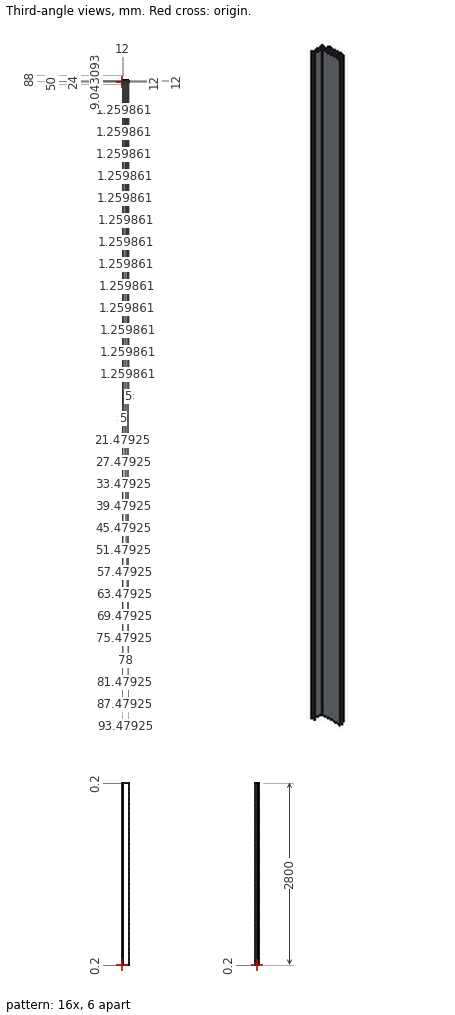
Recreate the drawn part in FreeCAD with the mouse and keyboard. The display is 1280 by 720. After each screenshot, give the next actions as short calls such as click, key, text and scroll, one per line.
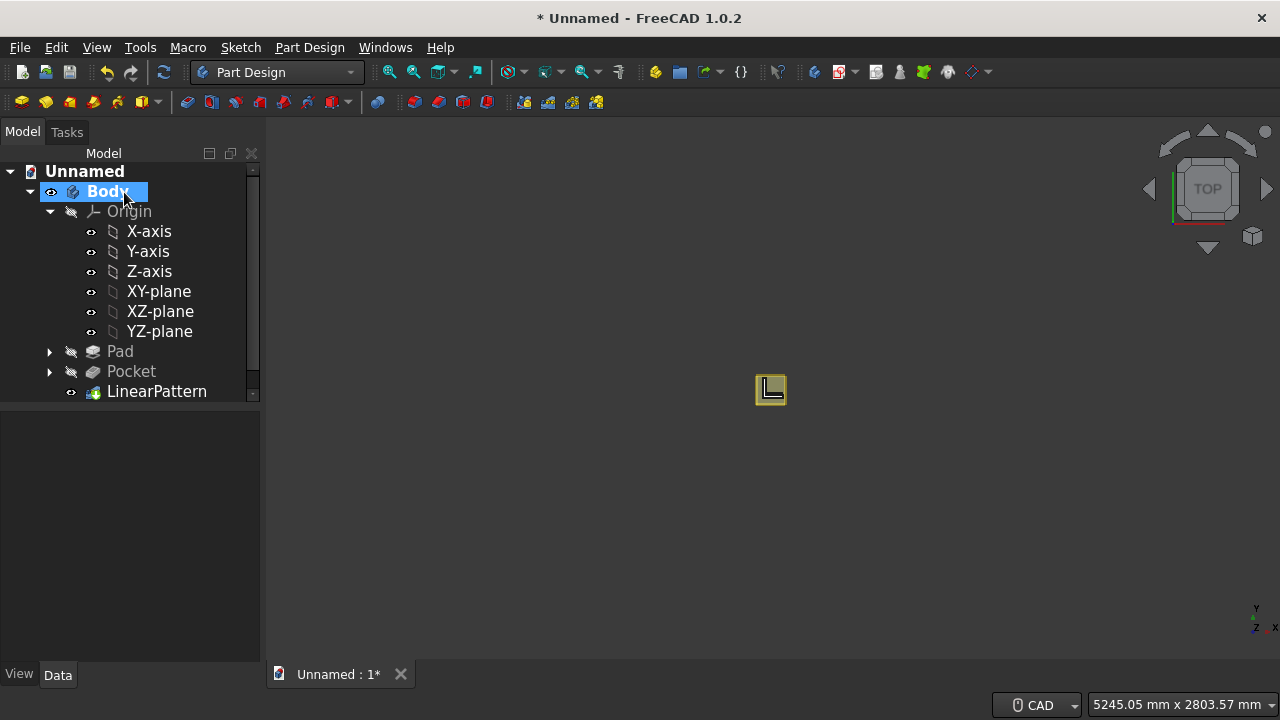
click(116, 372)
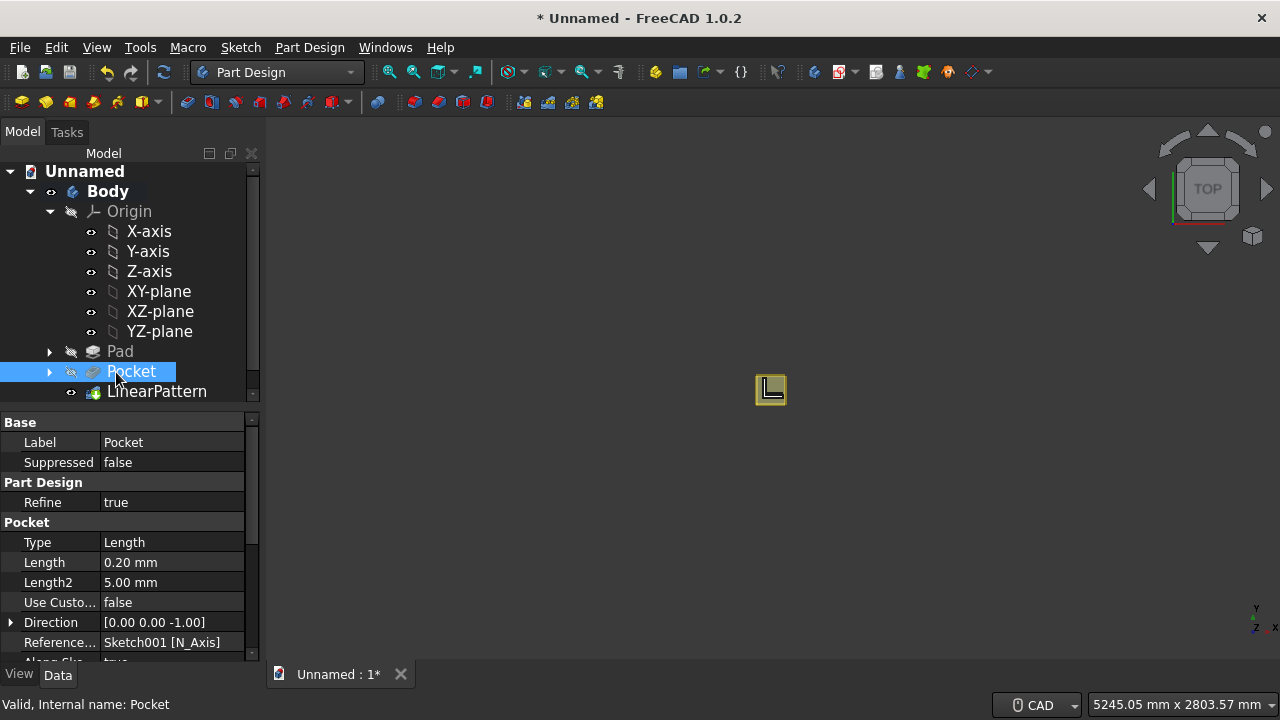
click(524, 102)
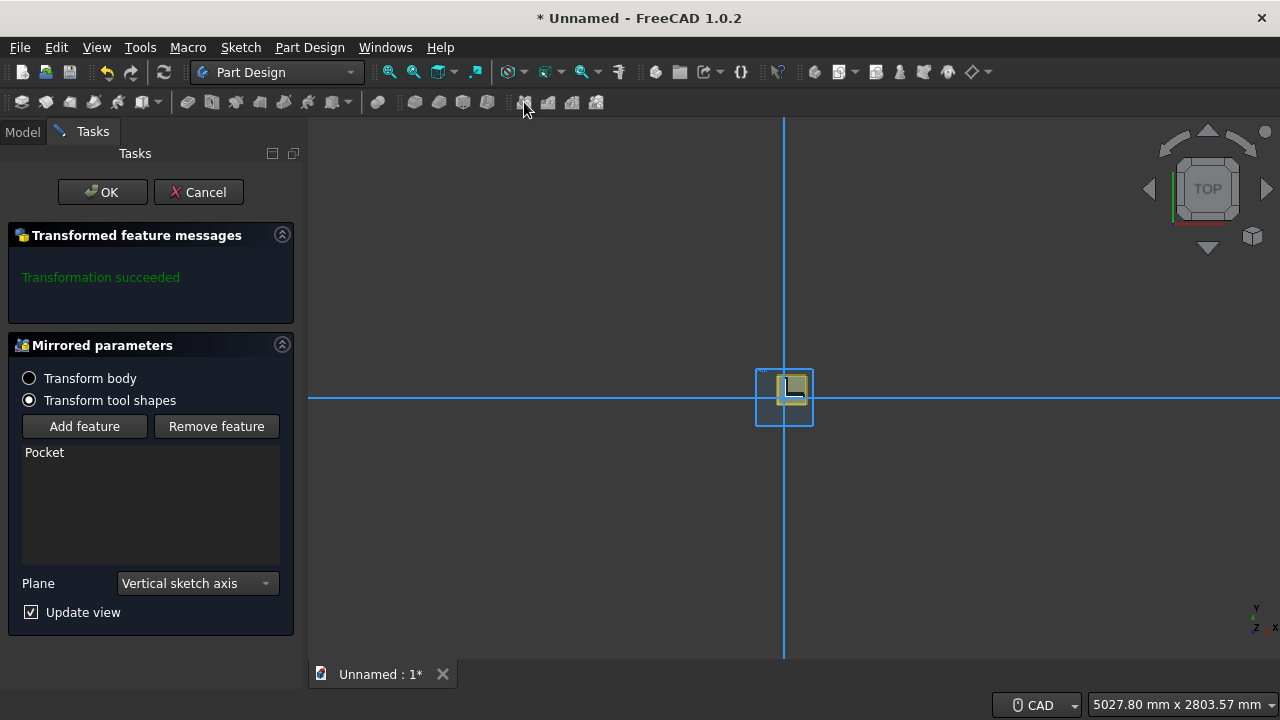
click(198, 584)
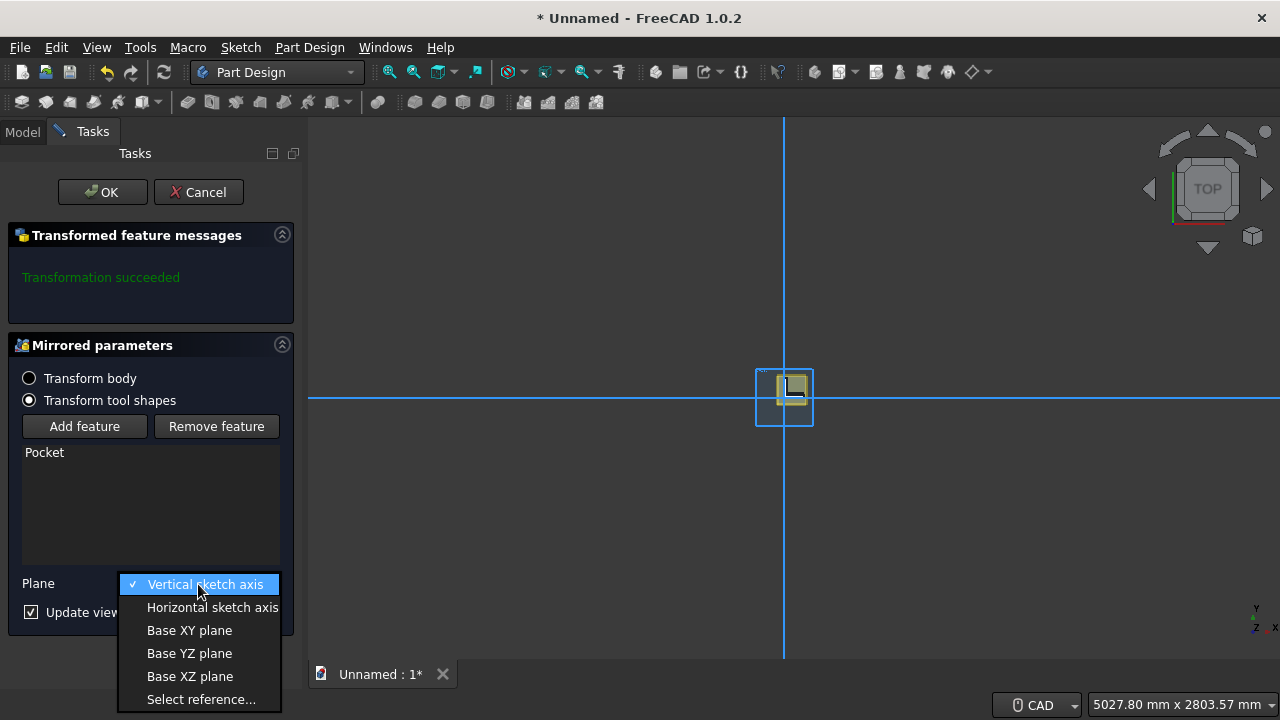
click(198, 700)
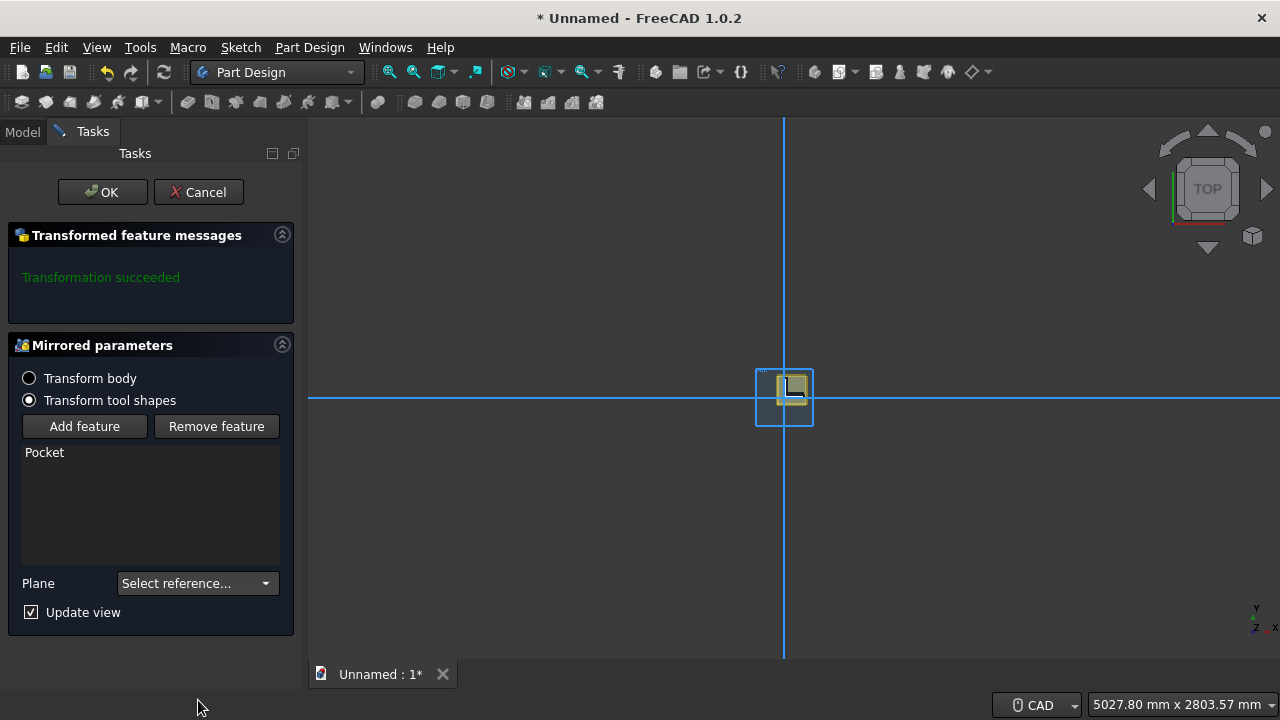
click(23, 131)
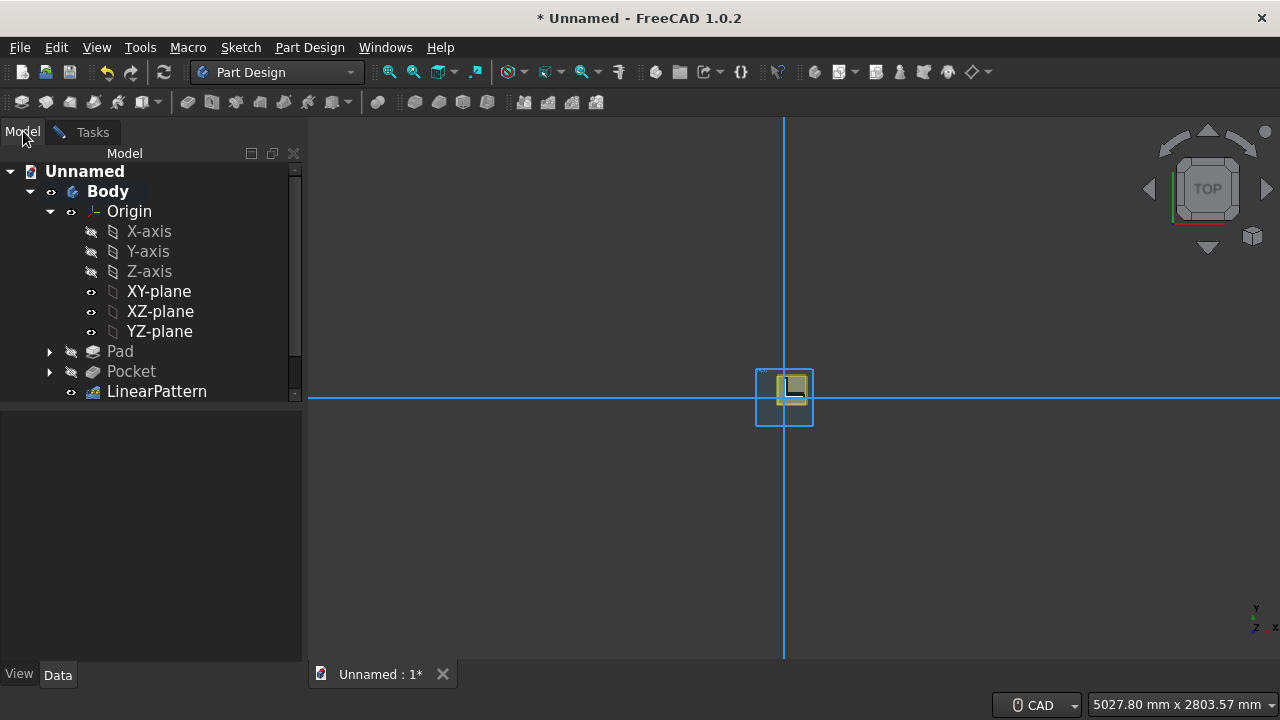
scroll(100, 287, down, 3)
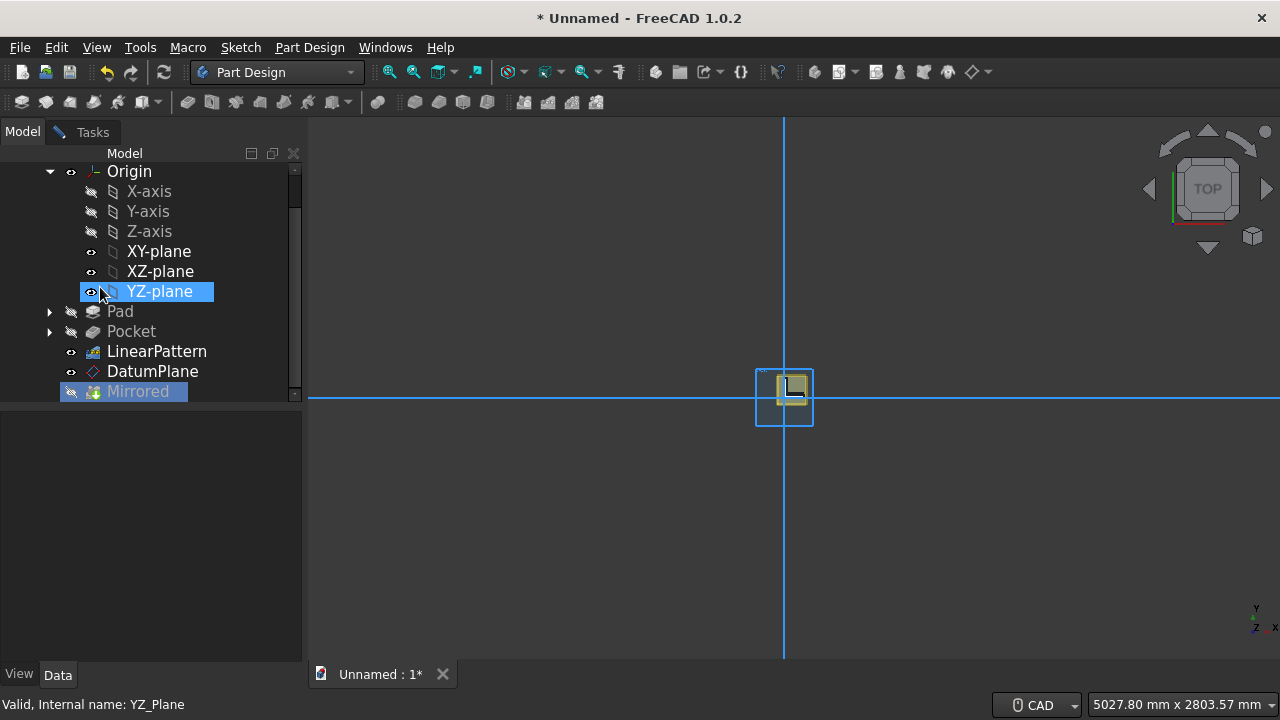
click(116, 372)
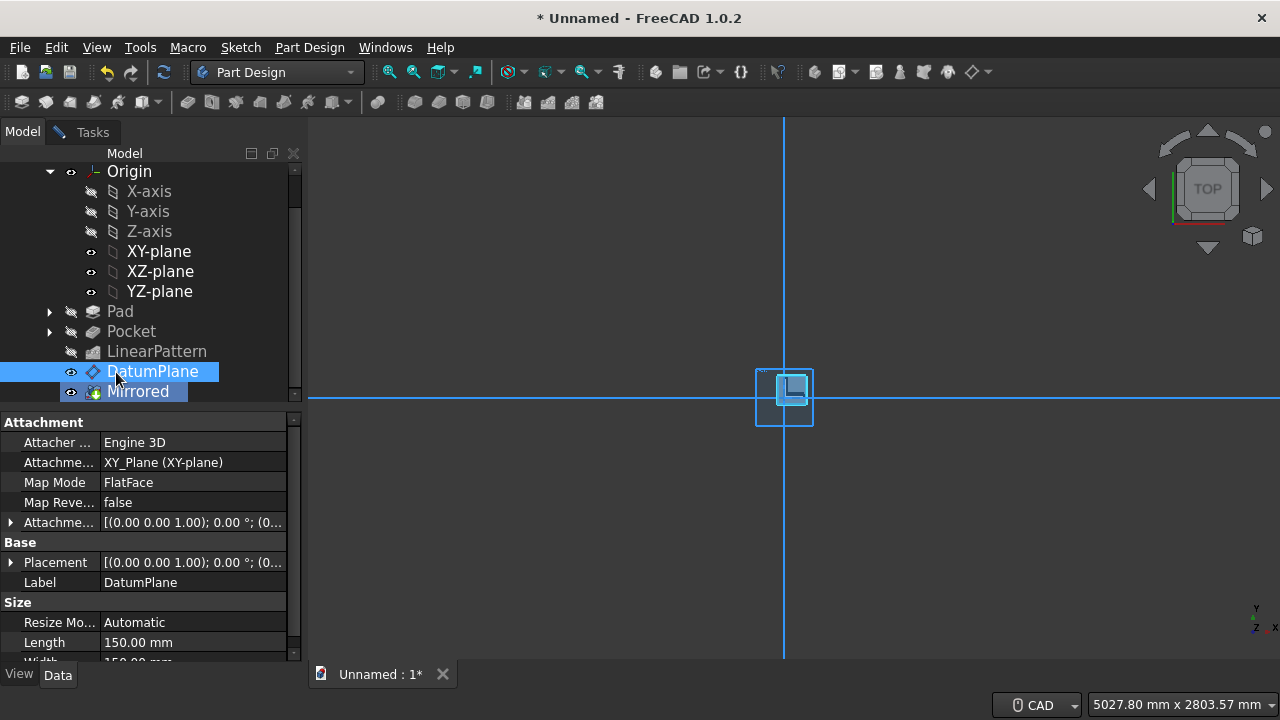
click(84, 131)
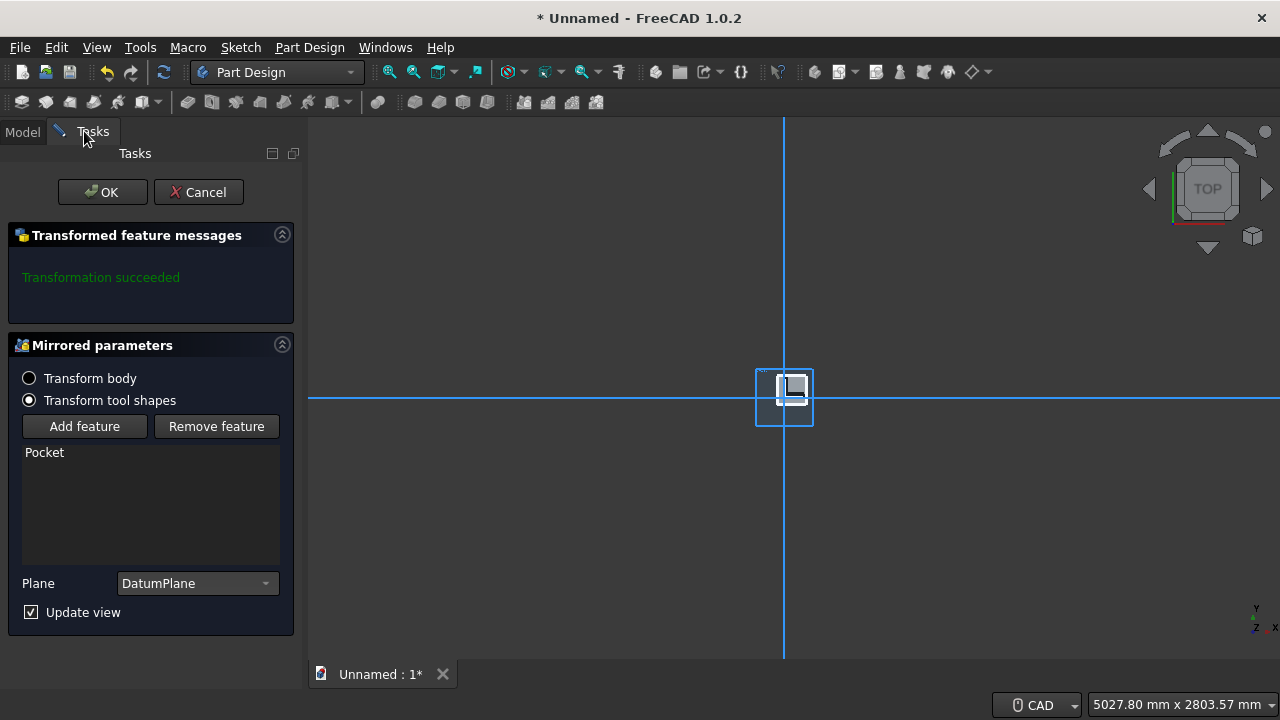
click(103, 192)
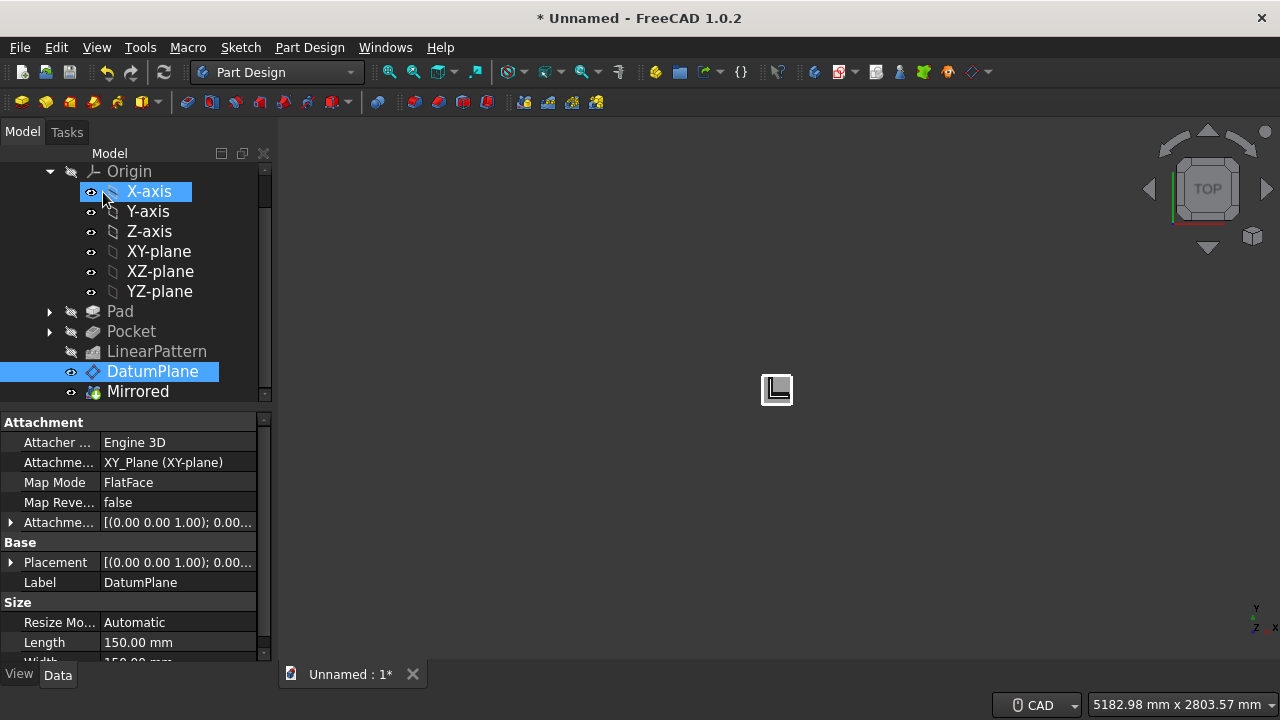
click(116, 372)
key(space)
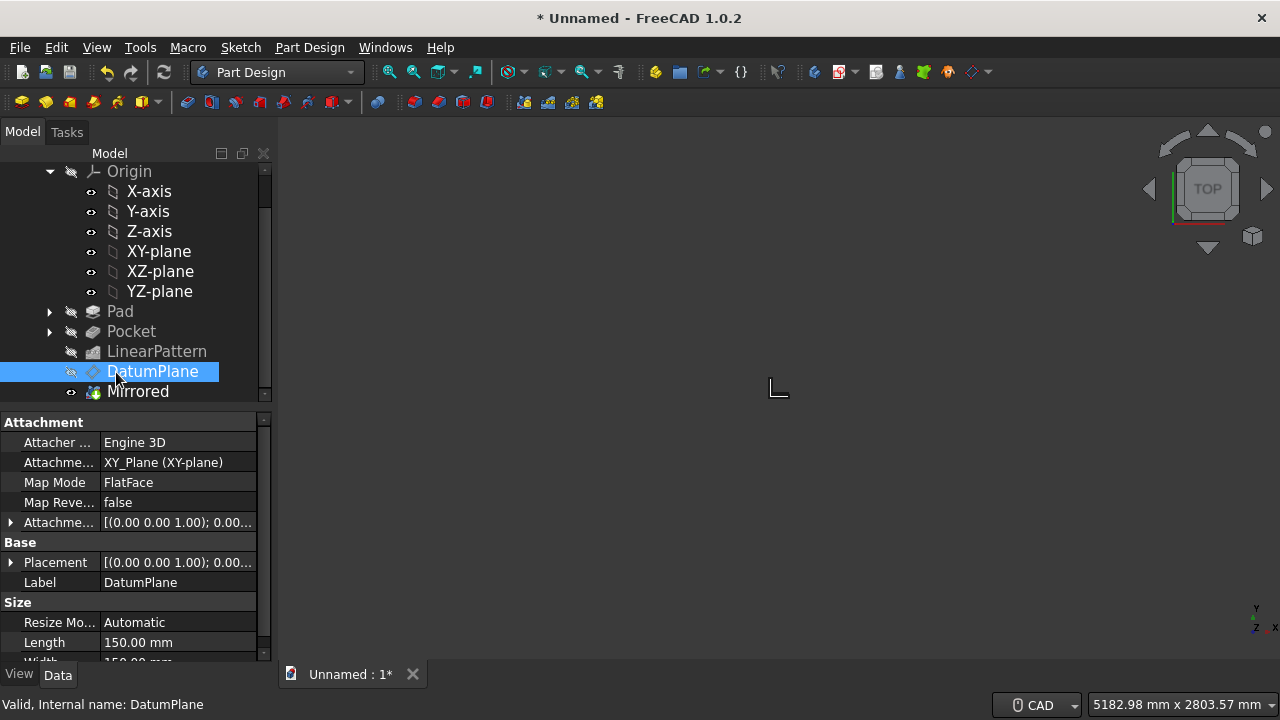
click(390, 72)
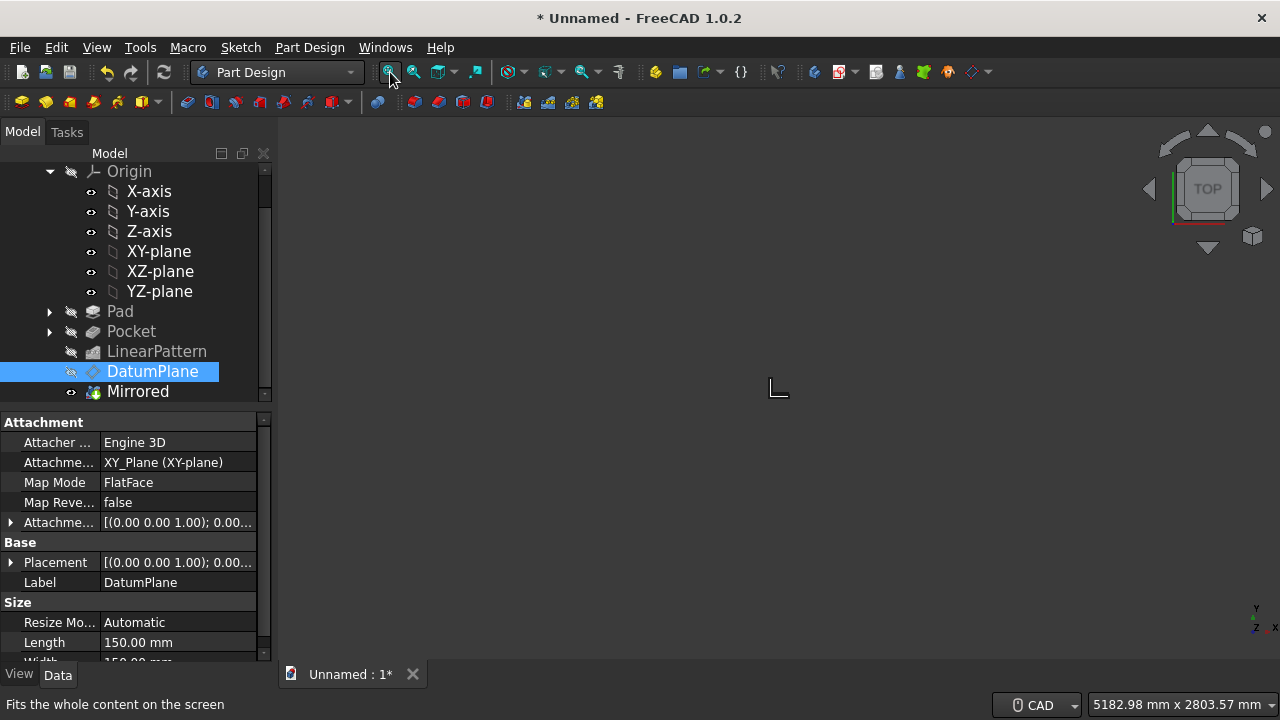
click(318, 619)